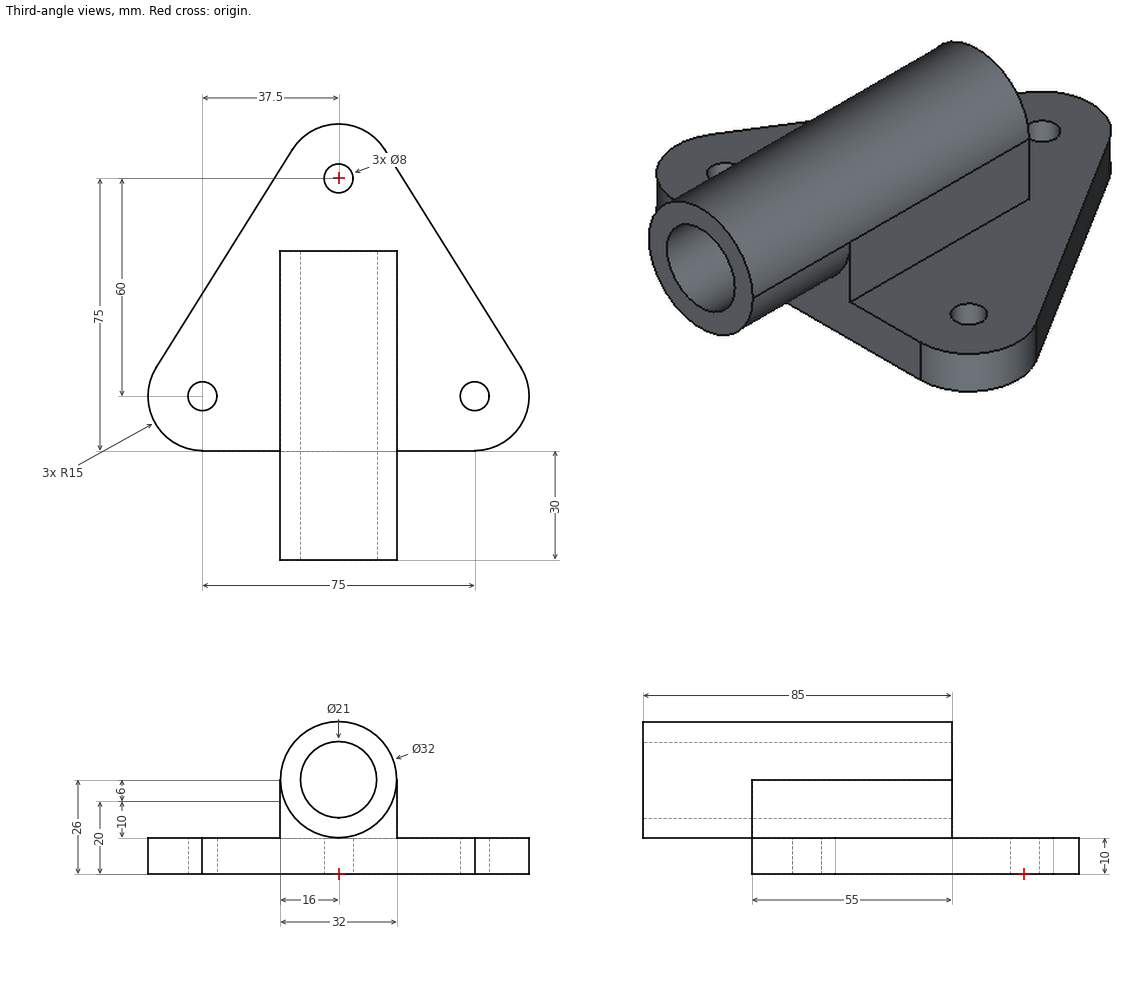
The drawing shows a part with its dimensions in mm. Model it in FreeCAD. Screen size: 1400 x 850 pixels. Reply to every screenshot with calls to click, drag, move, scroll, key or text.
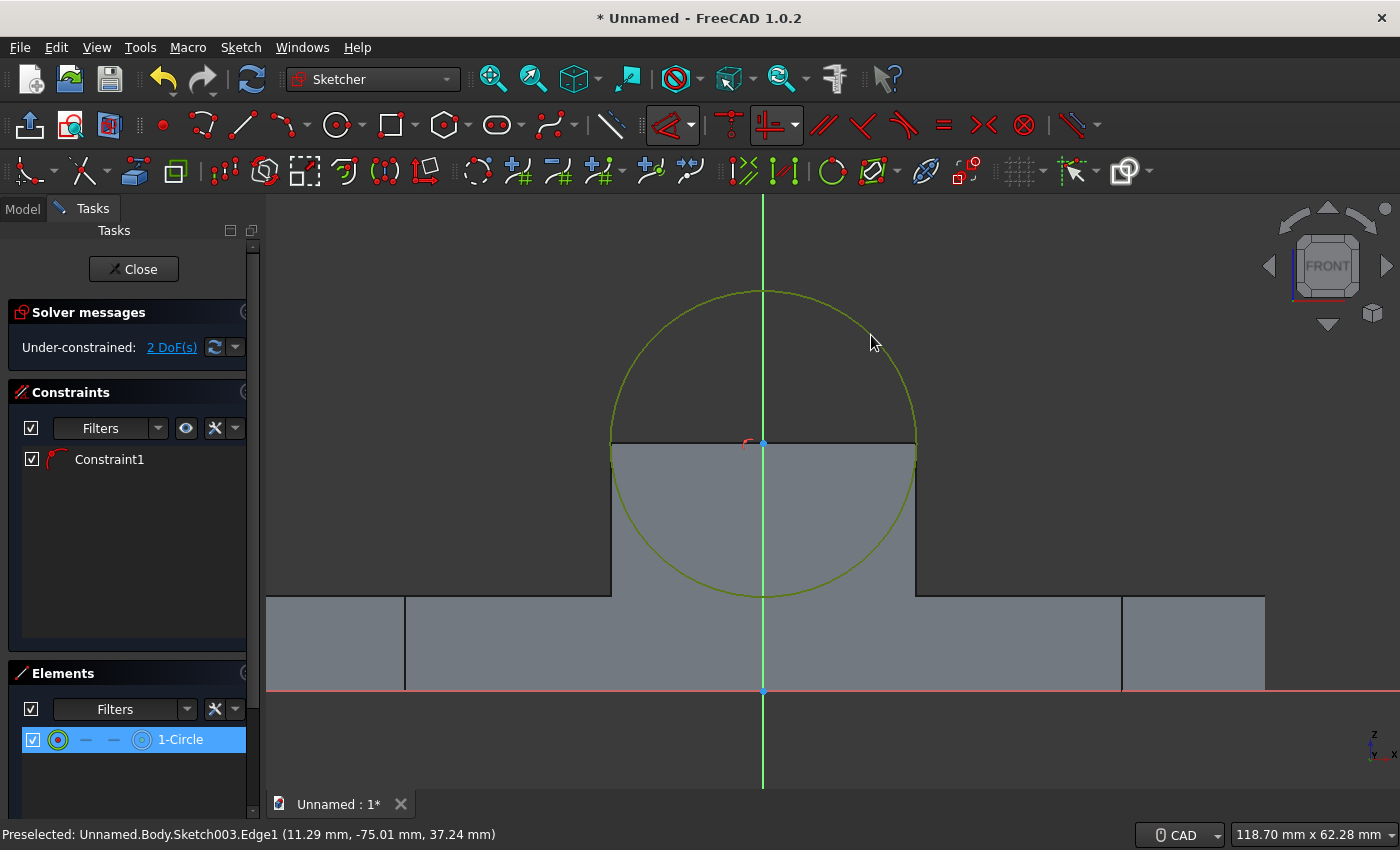
key(k)
key(o)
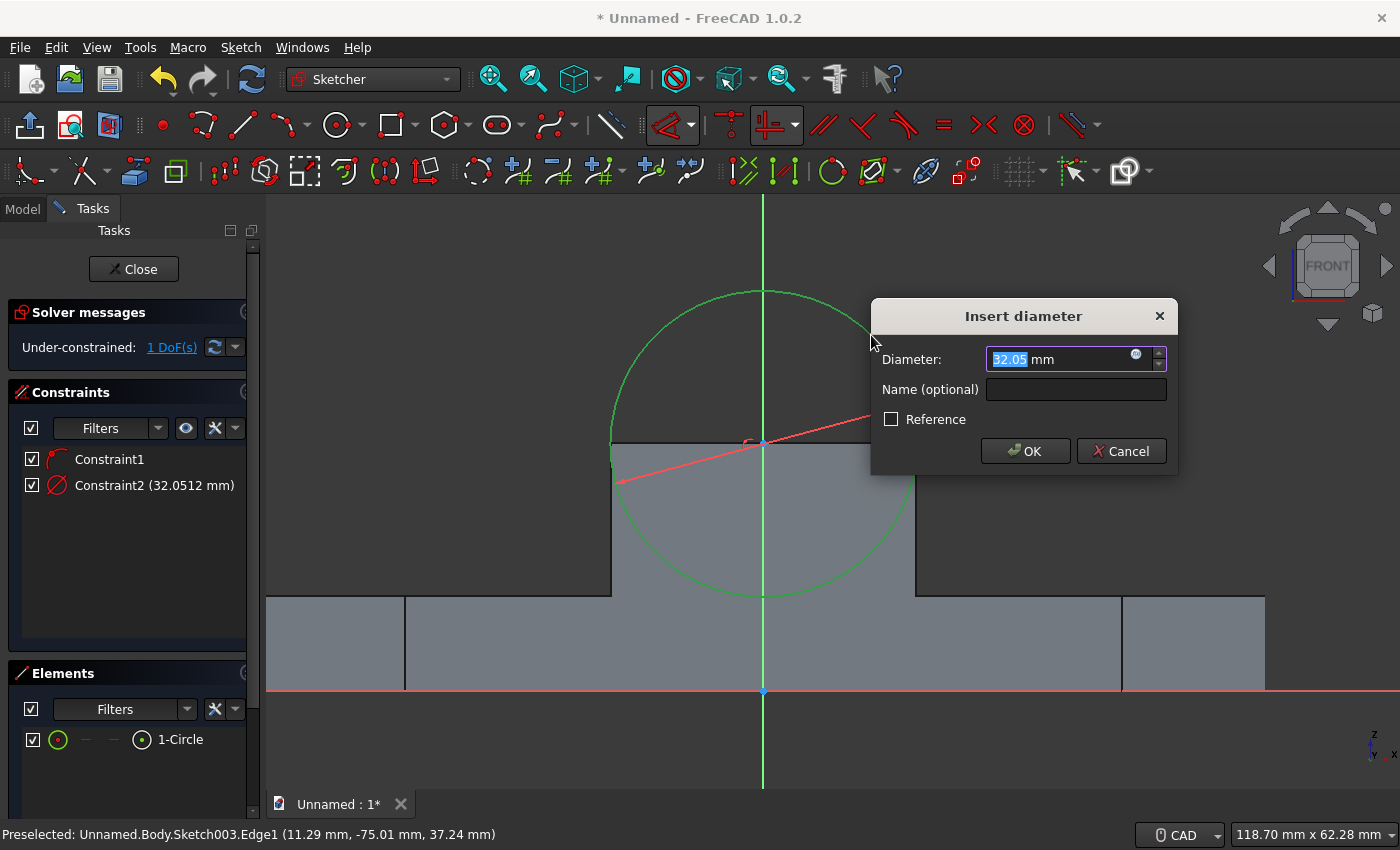
text(32)
key(Return)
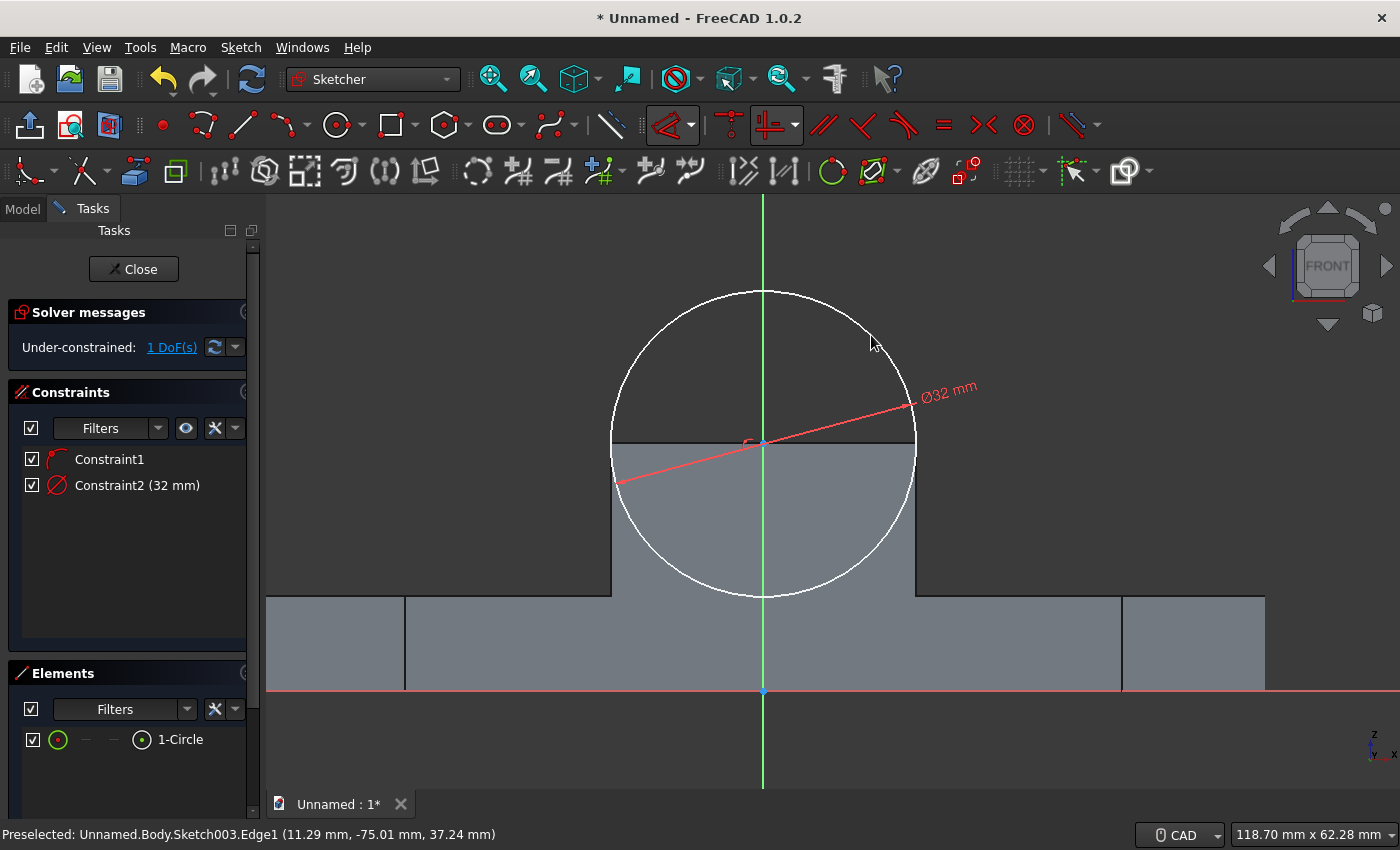
click(763, 444)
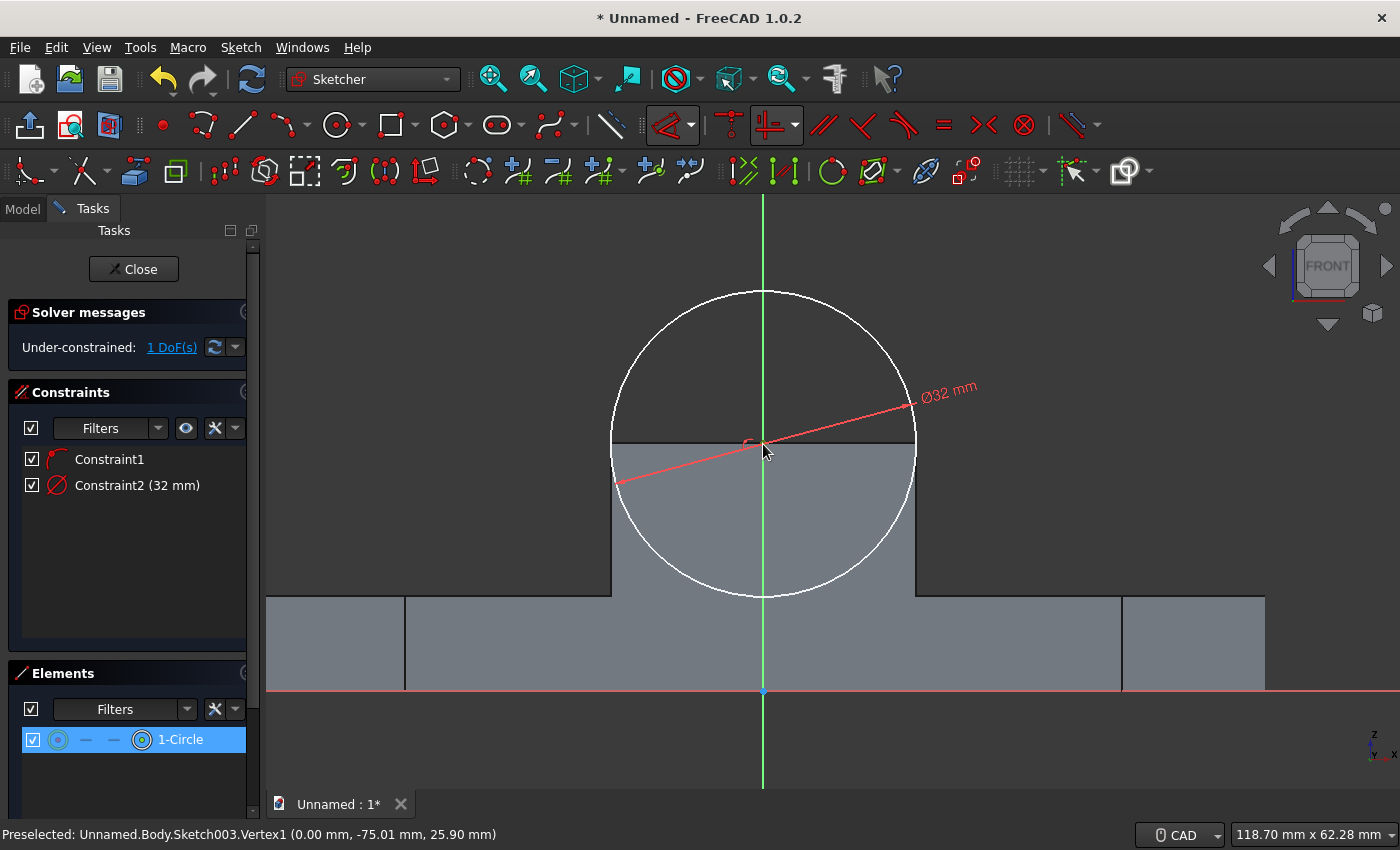
key(i)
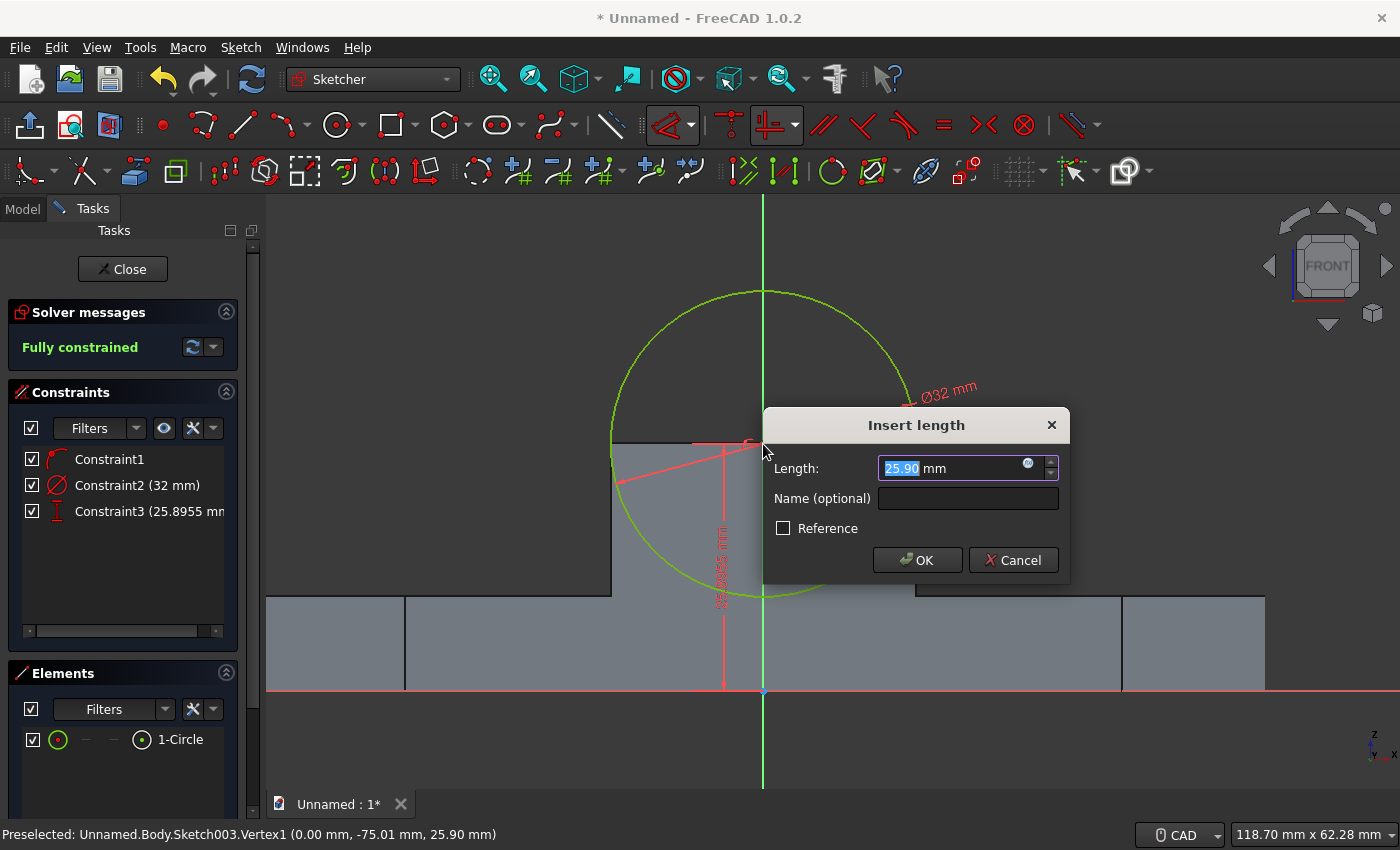
text(26)
key(Return)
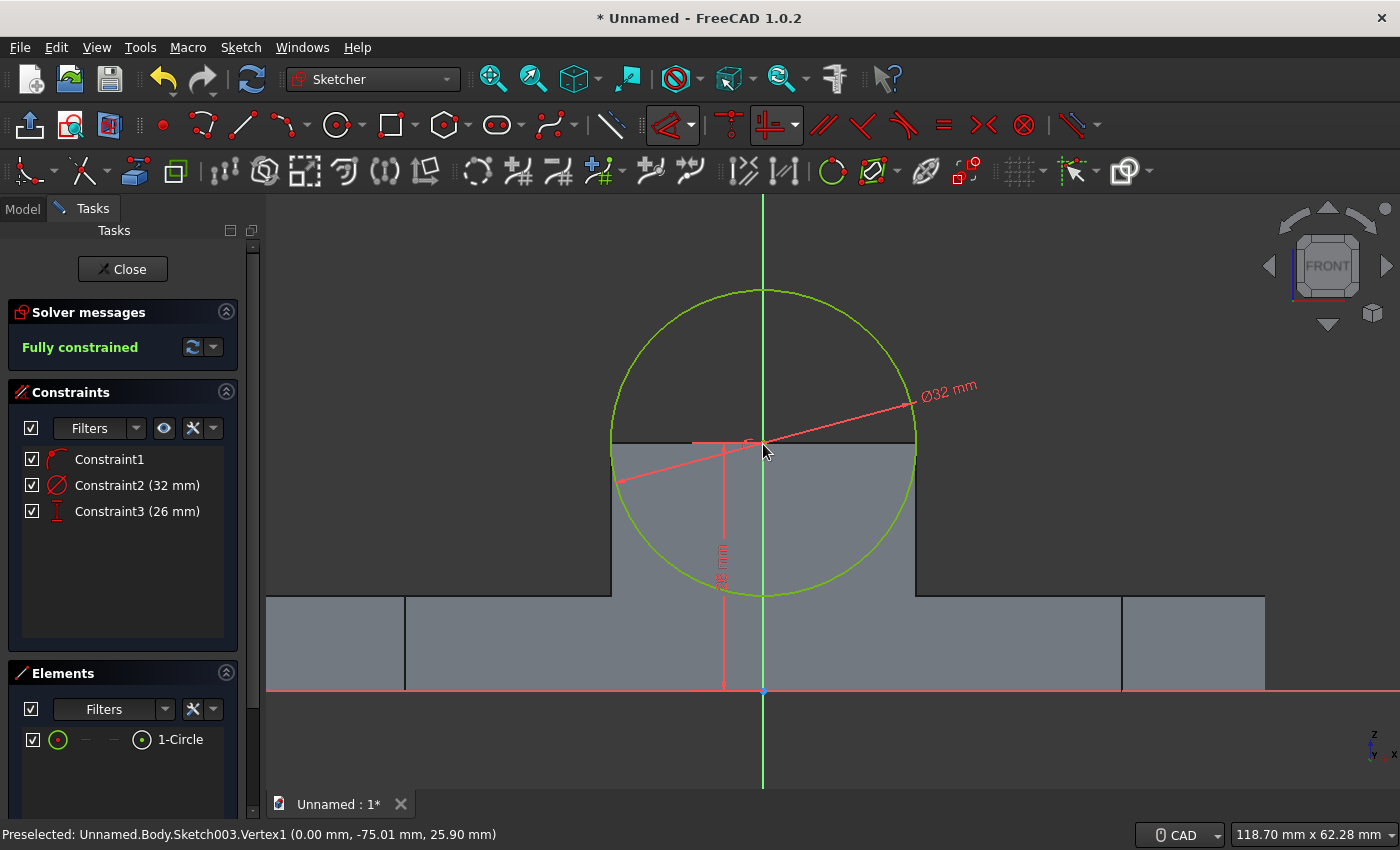
click(123, 269)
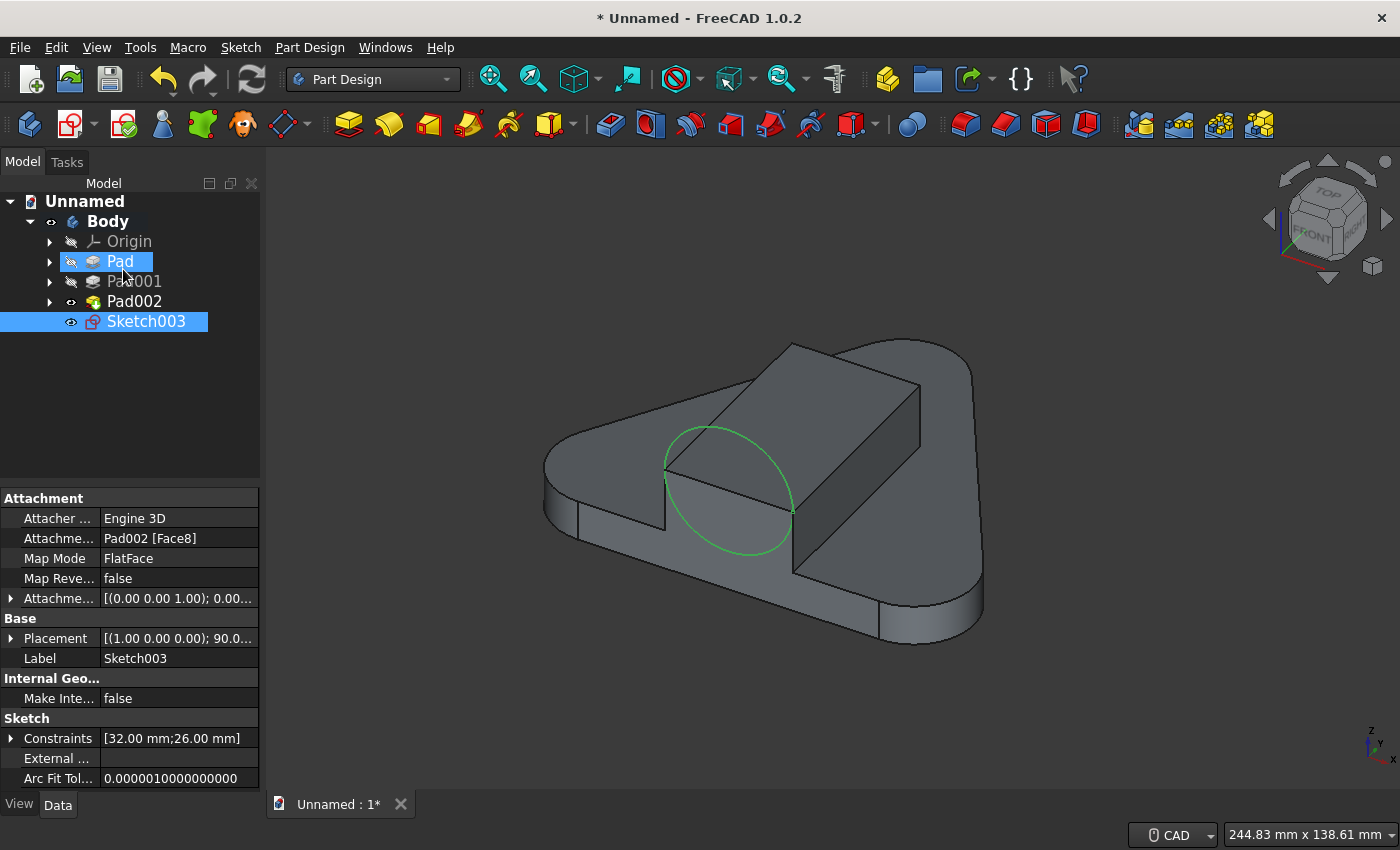
click(350, 124)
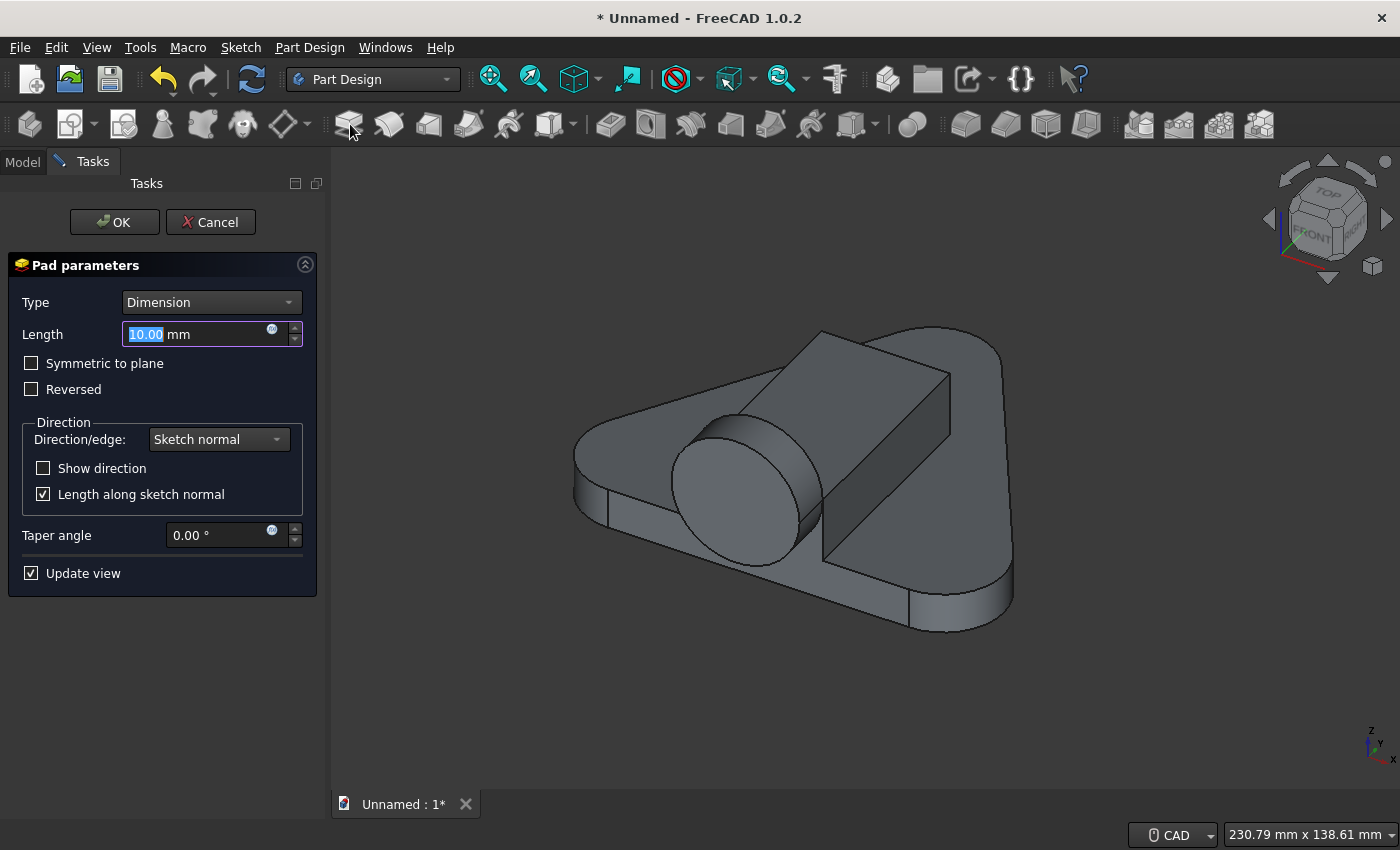
text(55)
key(Tab)